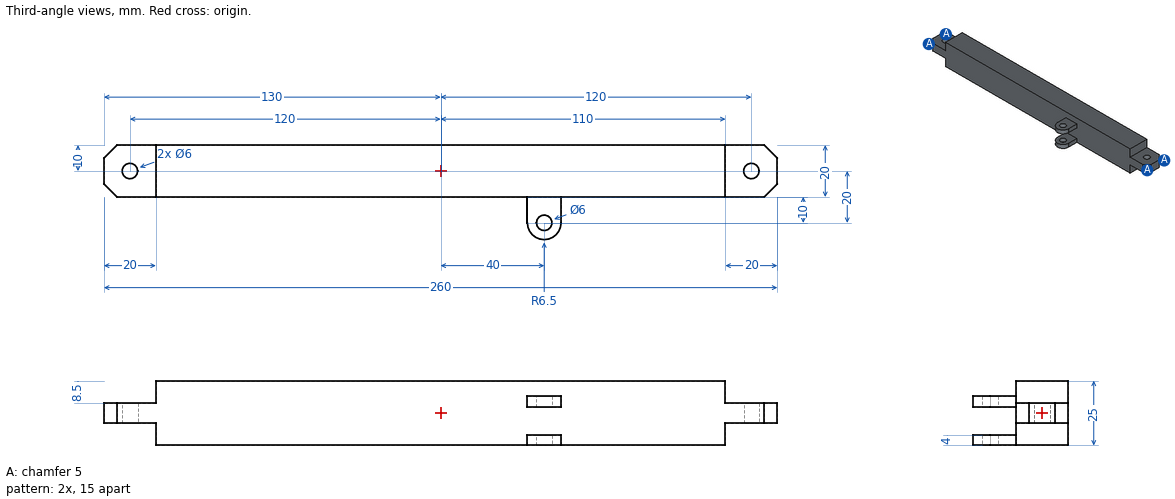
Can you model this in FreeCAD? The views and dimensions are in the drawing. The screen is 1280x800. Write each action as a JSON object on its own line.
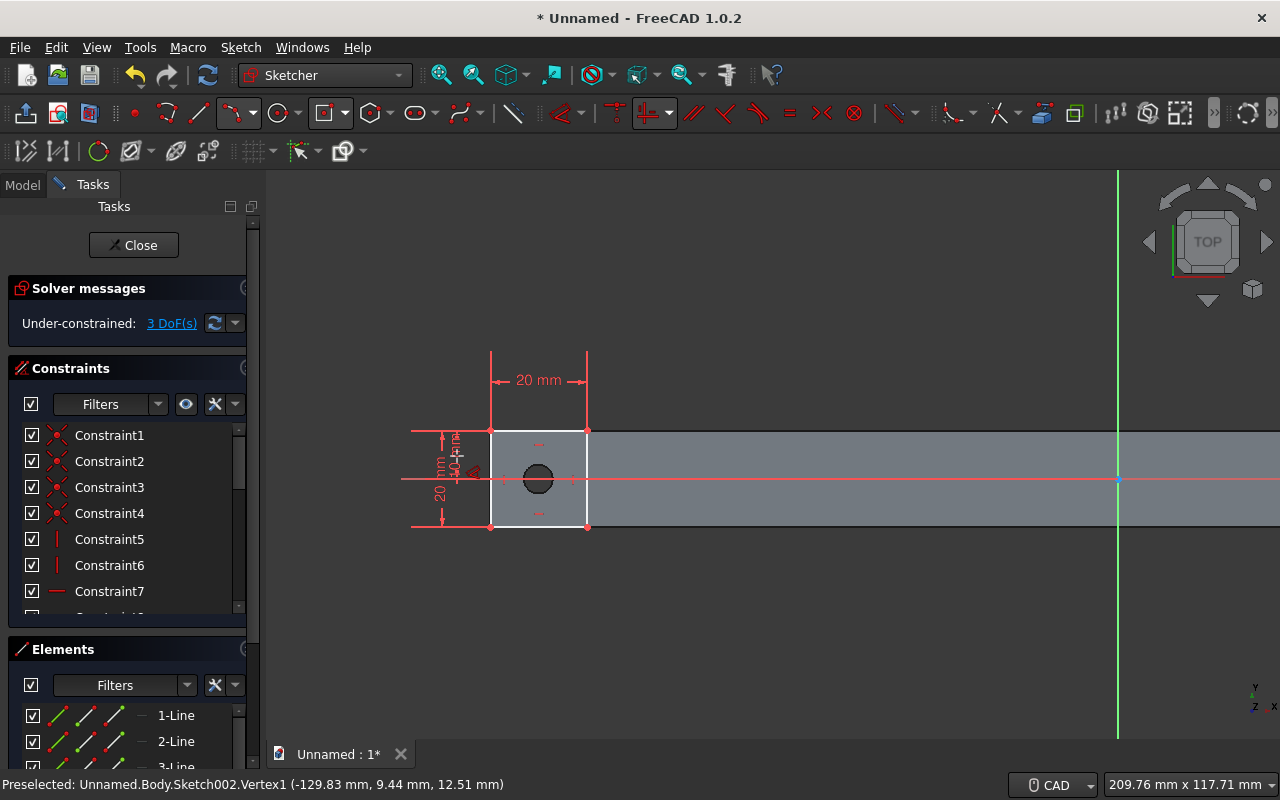
{"action": "scroll", "coordinate": [367, 434], "scroll_direction": "down", "scroll_amount": 4}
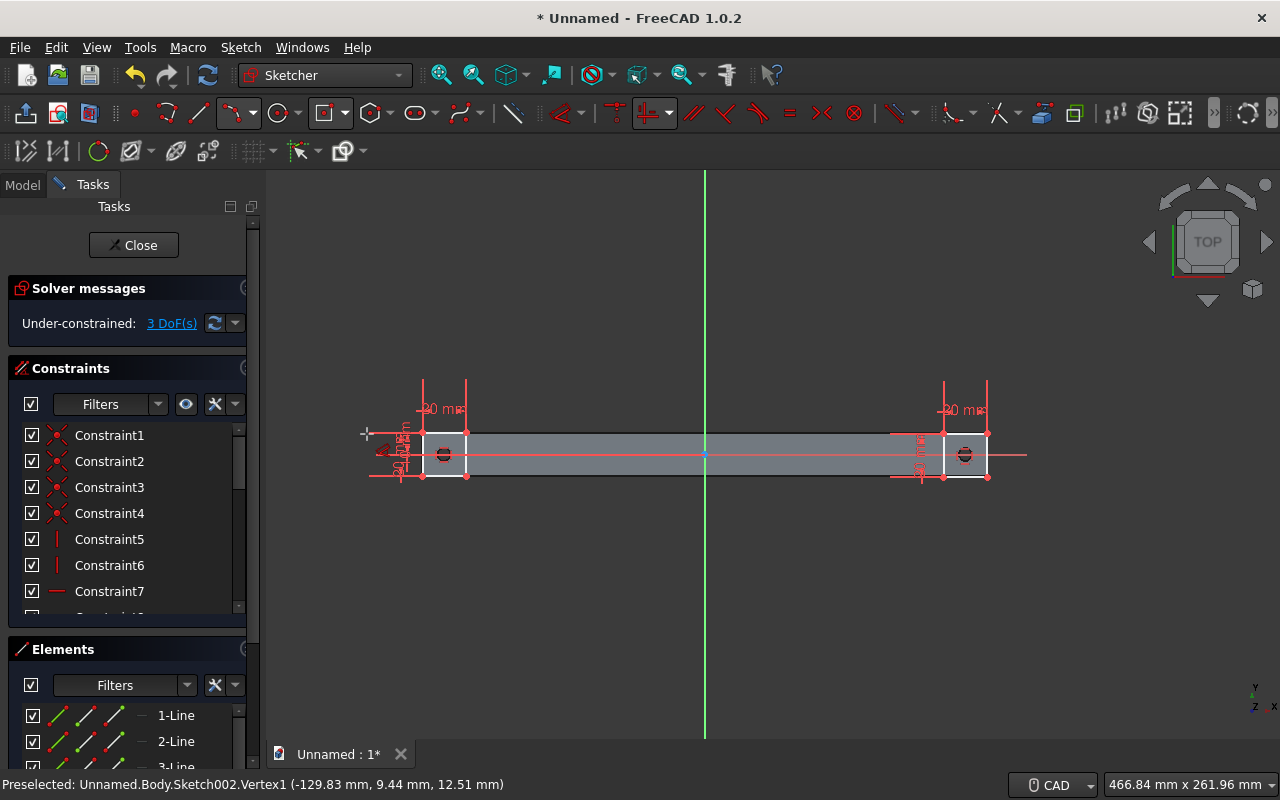
{"action": "scroll", "coordinate": [944, 434], "scroll_direction": "up", "scroll_amount": 4}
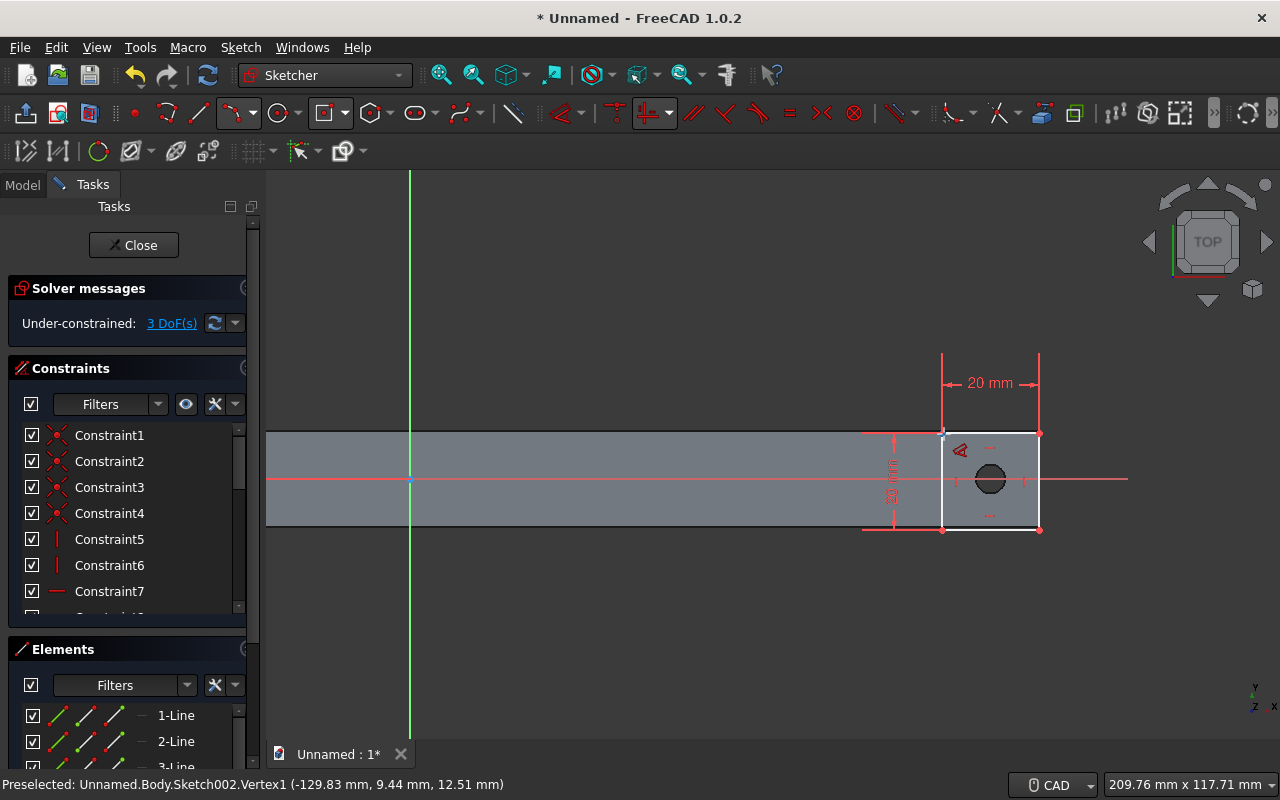
{"action": "left_click", "coordinate": [942, 433]}
{"action": "left_click", "coordinate": [976, 456]}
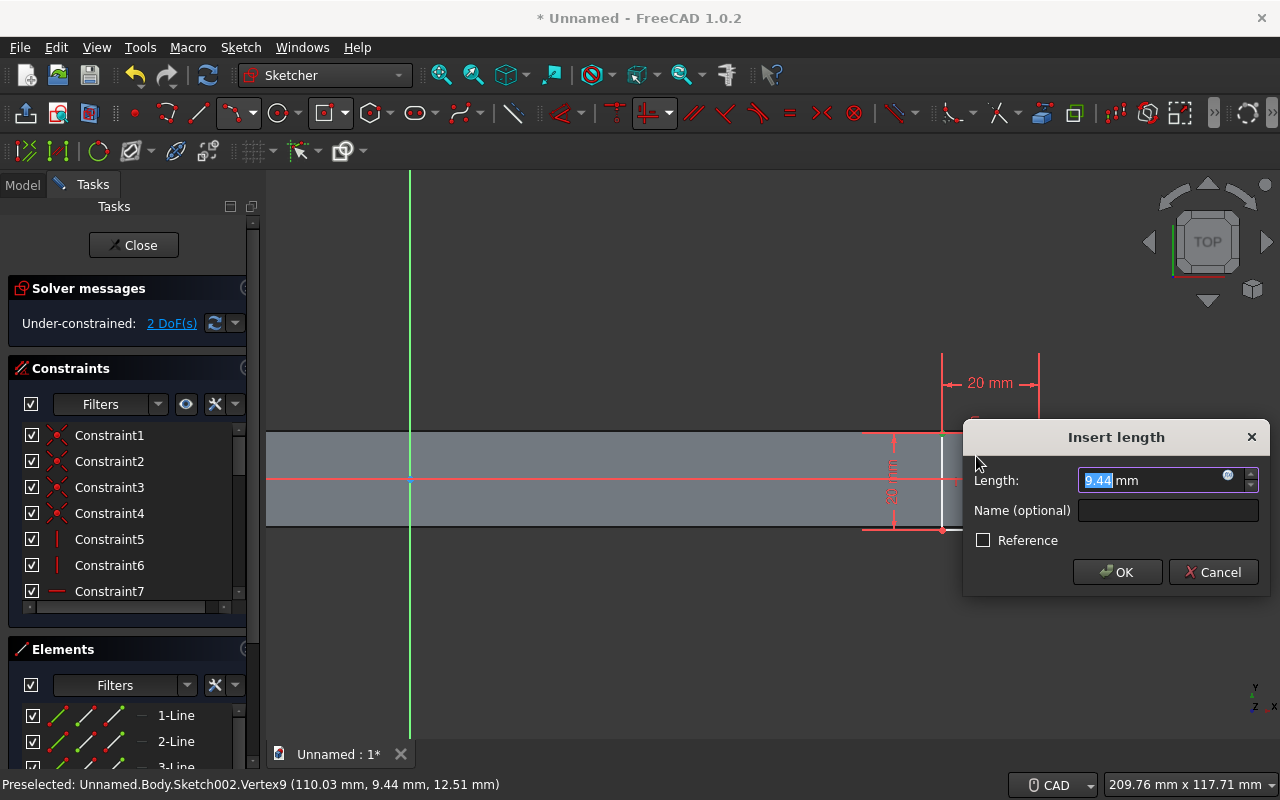
{"action": "type", "text": "10"}
{"action": "key", "text": "Return"}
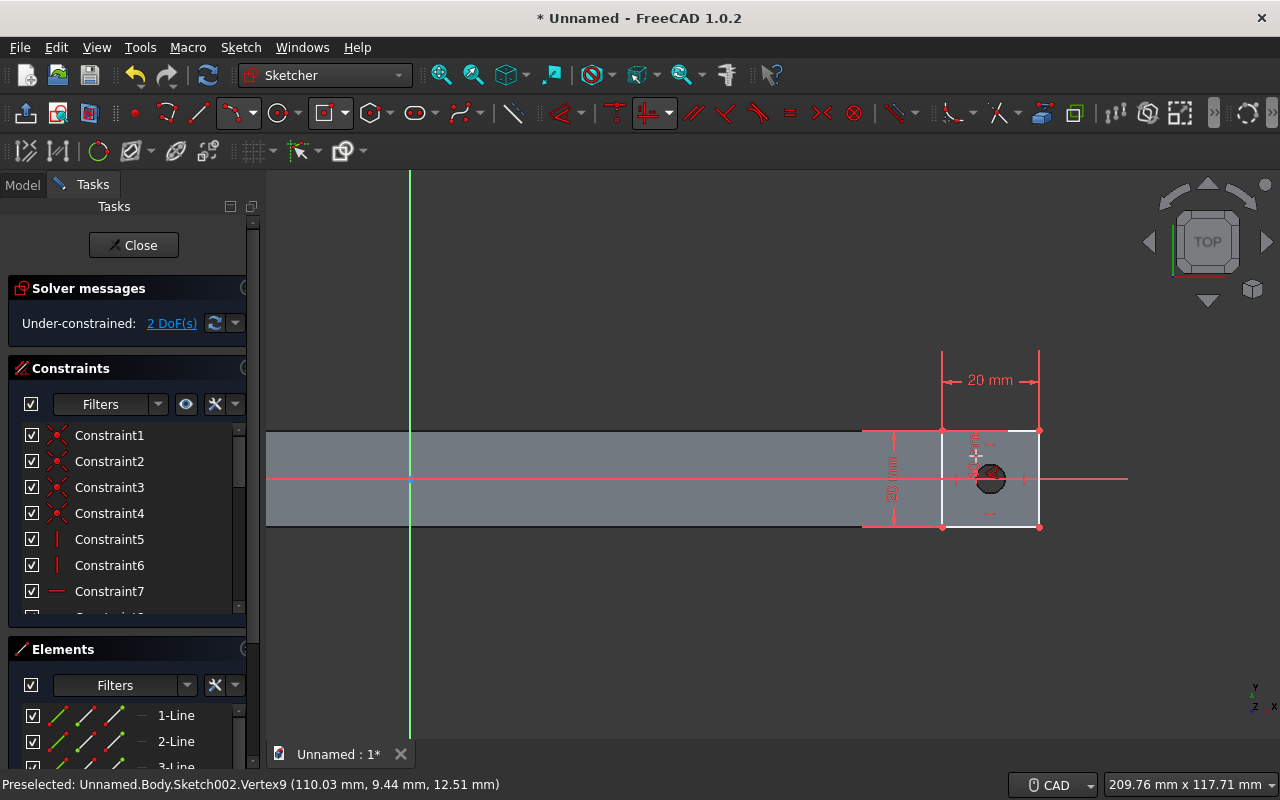
{"action": "scroll", "coordinate": [944, 434], "scroll_direction": "down", "scroll_amount": 4}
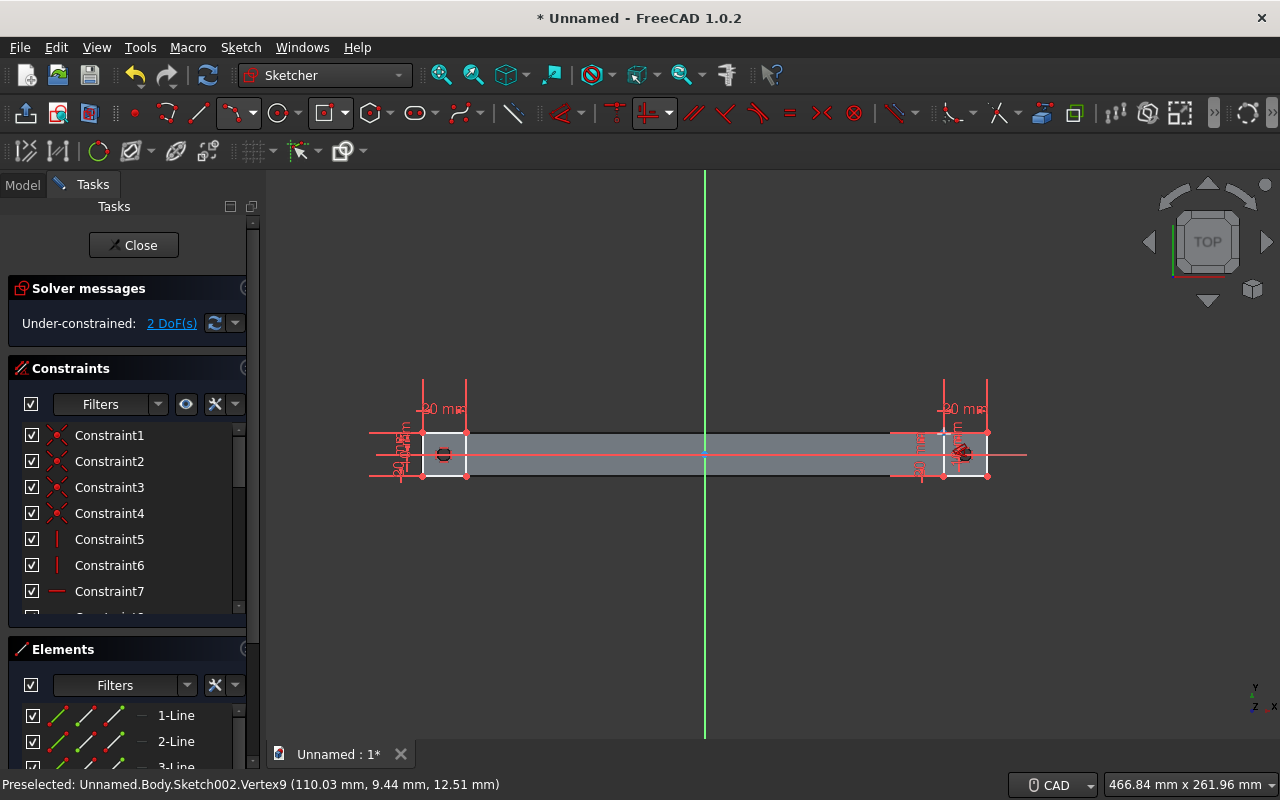
{"action": "left_click", "coordinate": [423, 433]}
{"action": "left_click", "coordinate": [564, 399]}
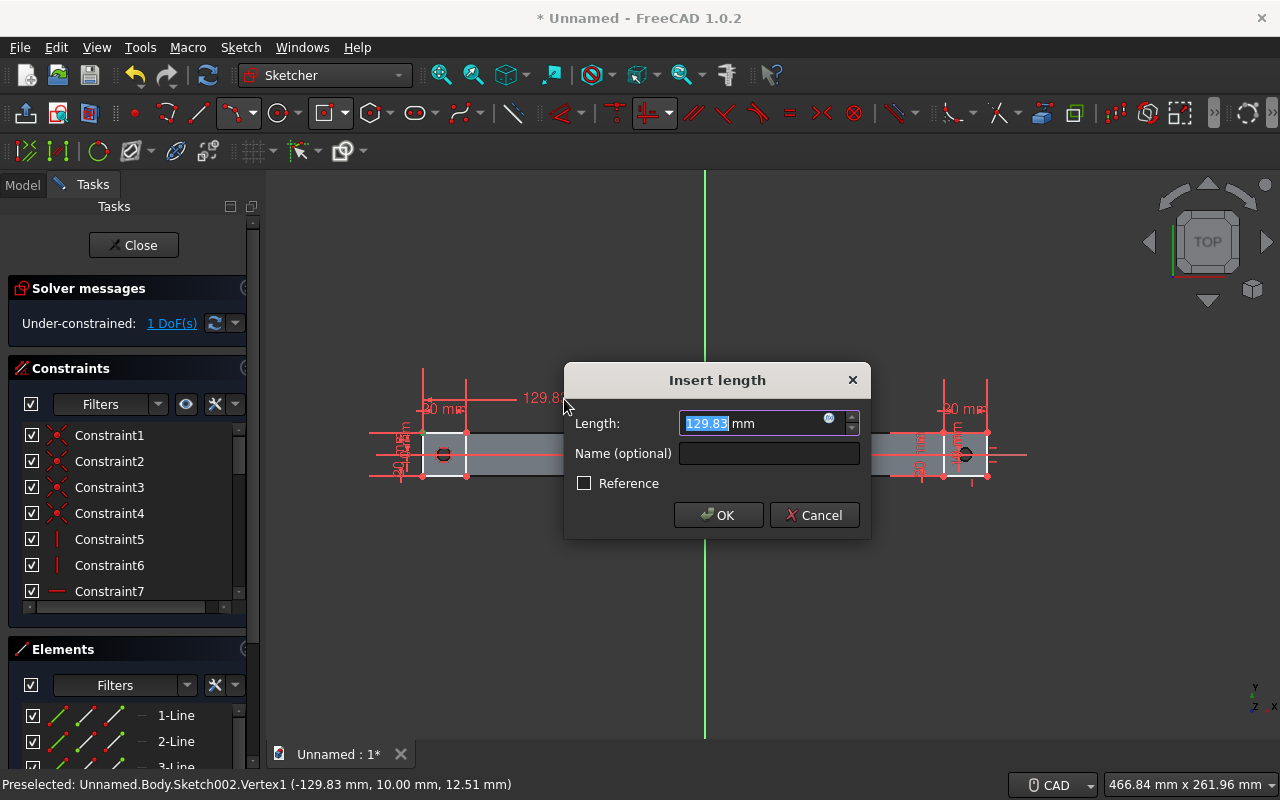
{"action": "type", "text": "130"}
{"action": "key", "text": "Return"}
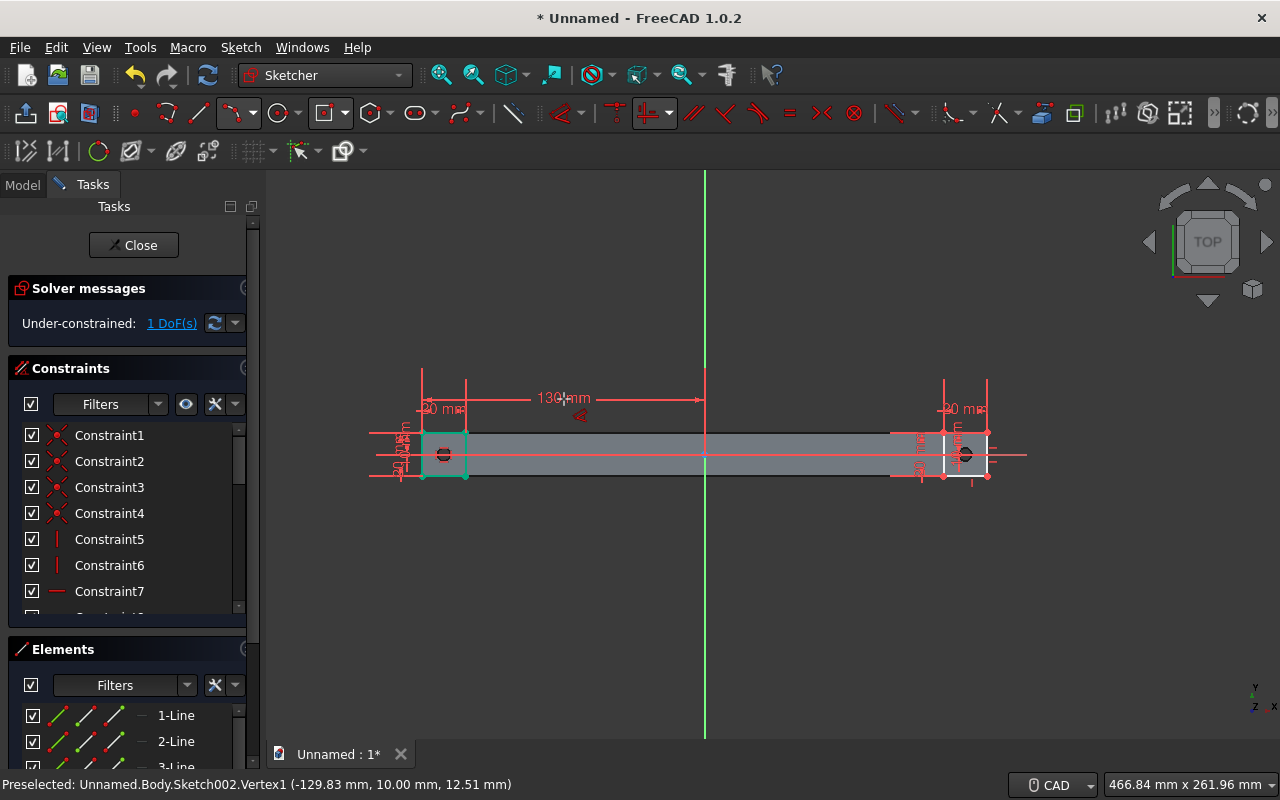
{"action": "left_click", "coordinate": [944, 433]}
{"action": "left_click", "coordinate": [824, 399]}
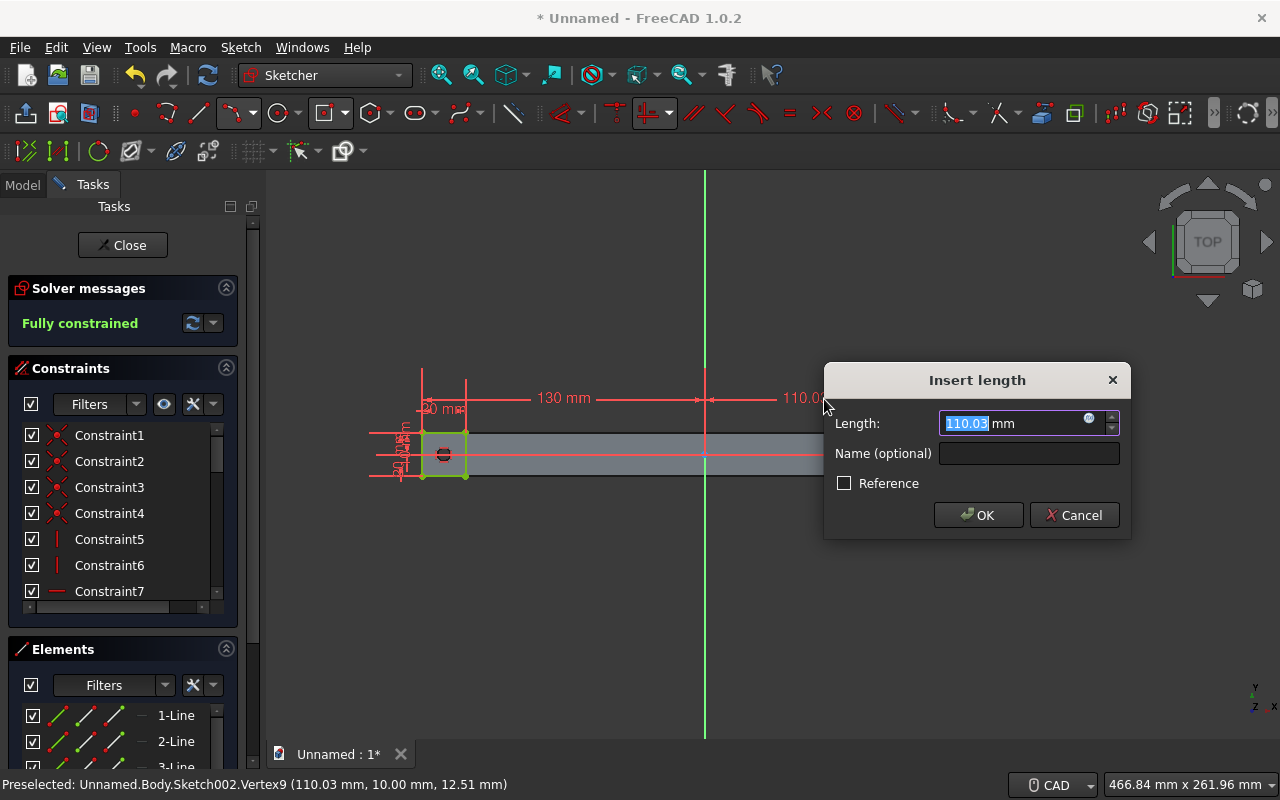
{"action": "type", "text": "110"}
{"action": "key", "text": "Return"}
{"action": "key", "text": "Escape"}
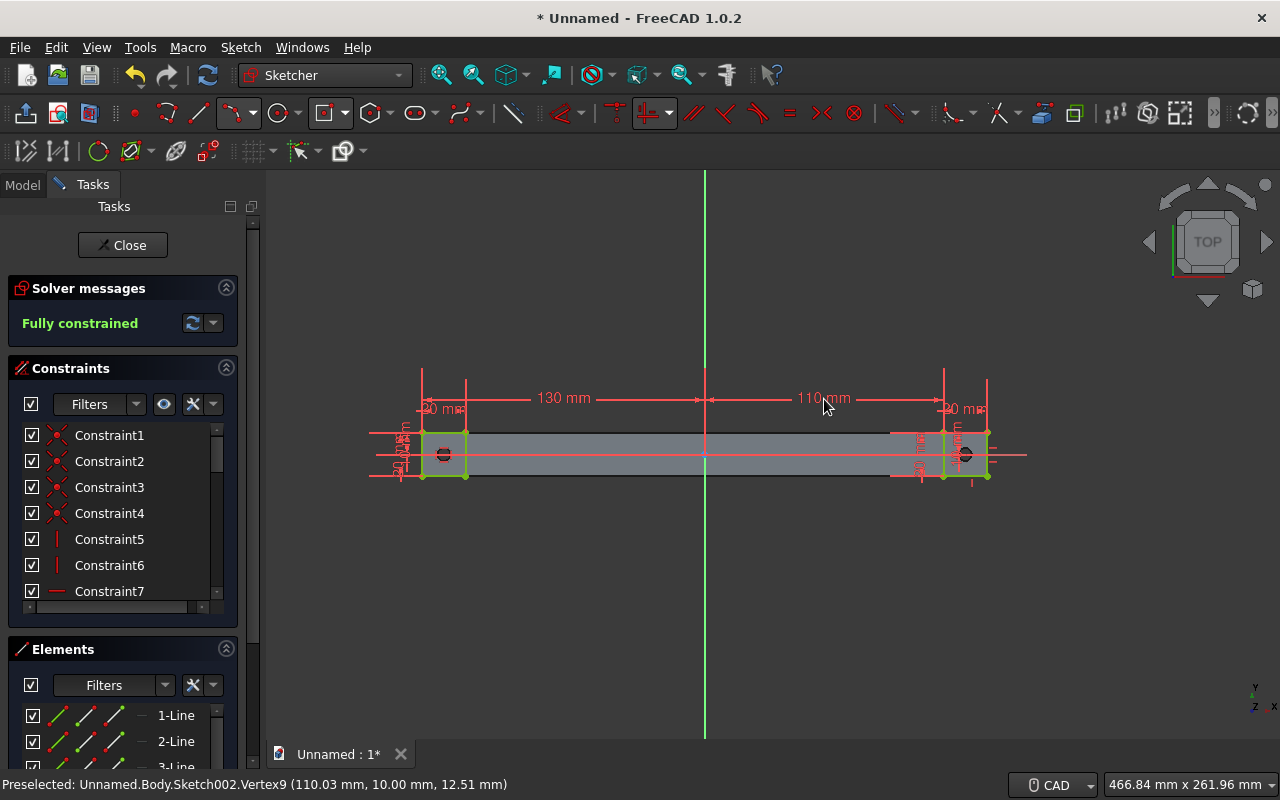
{"action": "left_click", "coordinate": [123, 245]}